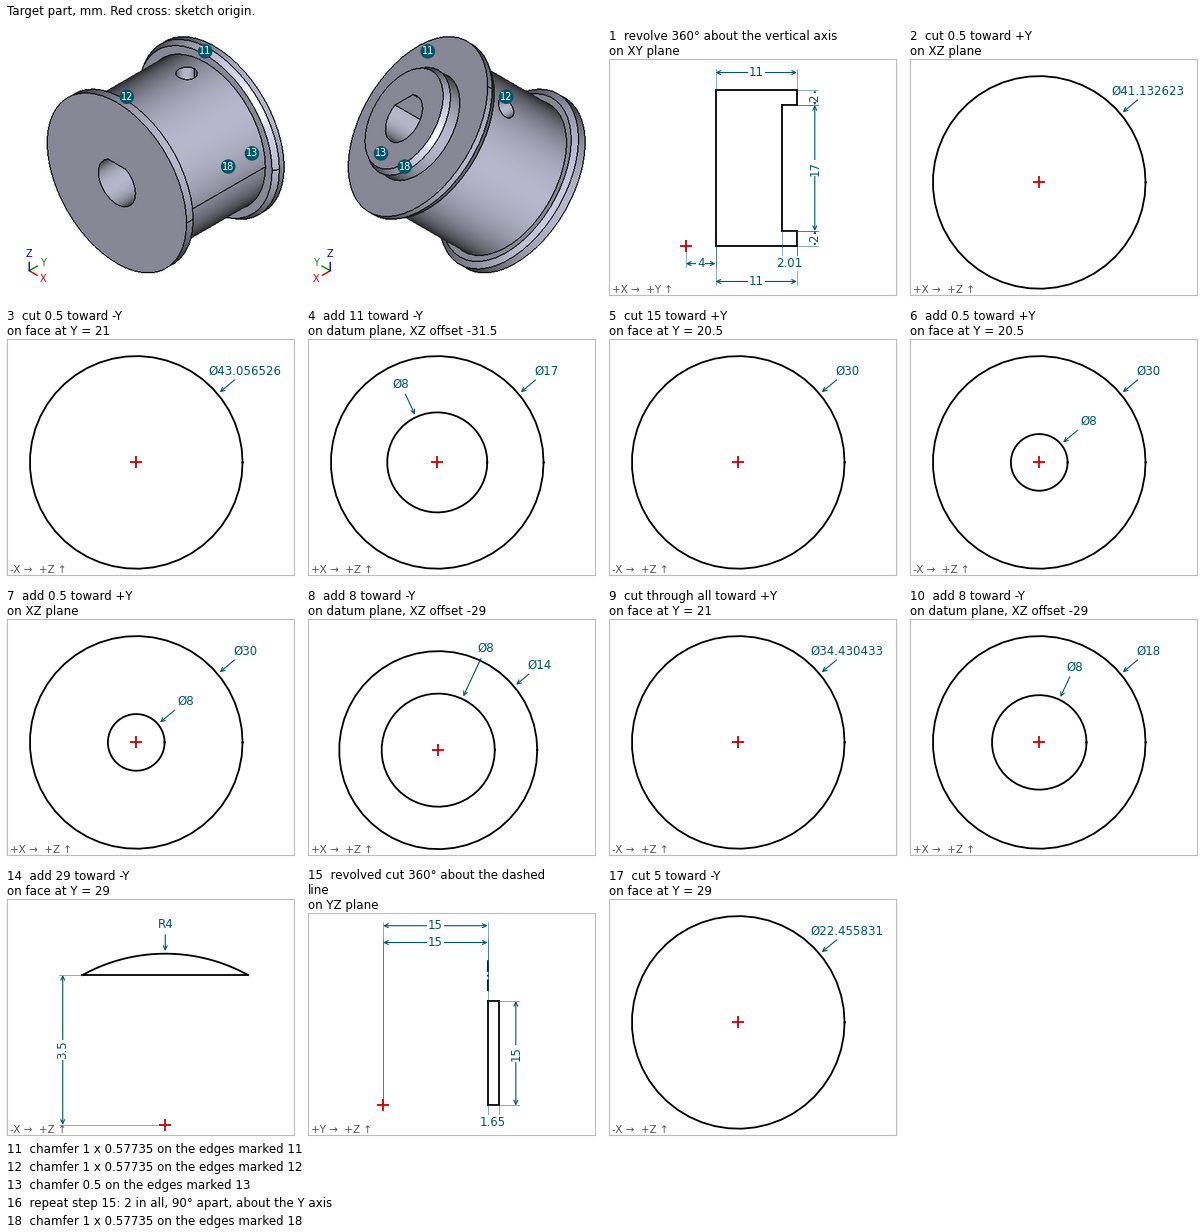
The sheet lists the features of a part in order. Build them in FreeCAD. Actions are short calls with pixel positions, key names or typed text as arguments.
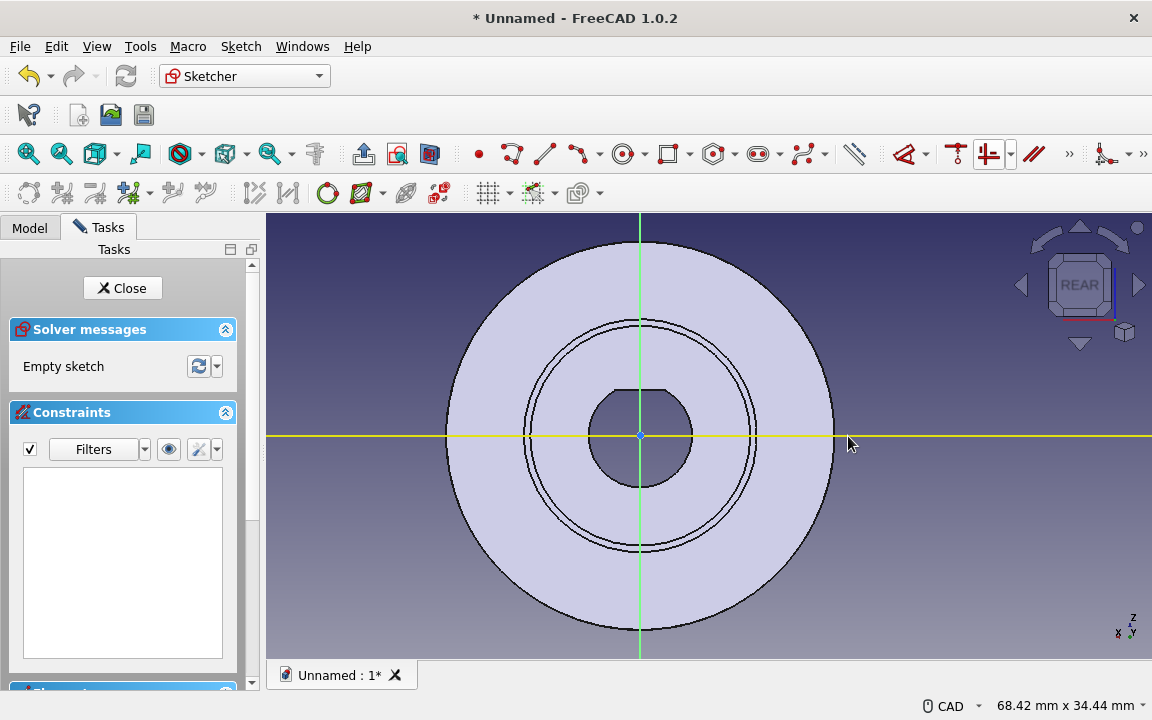
click(622, 154)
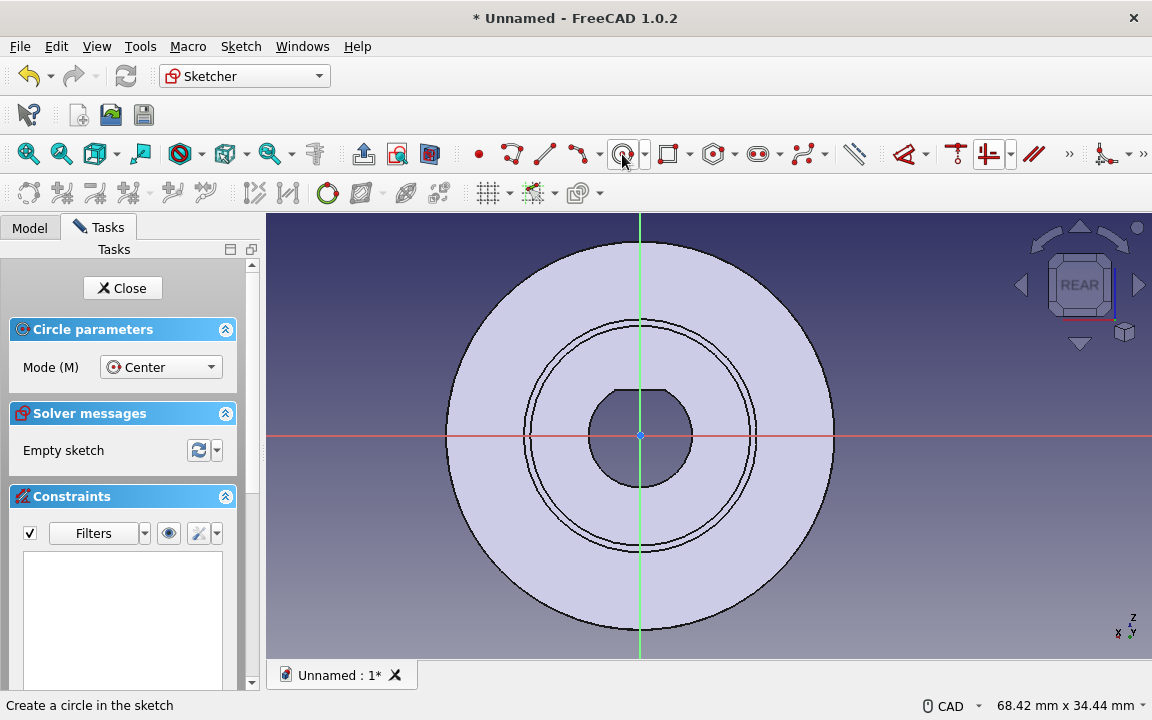
click(640, 436)
move(743, 333)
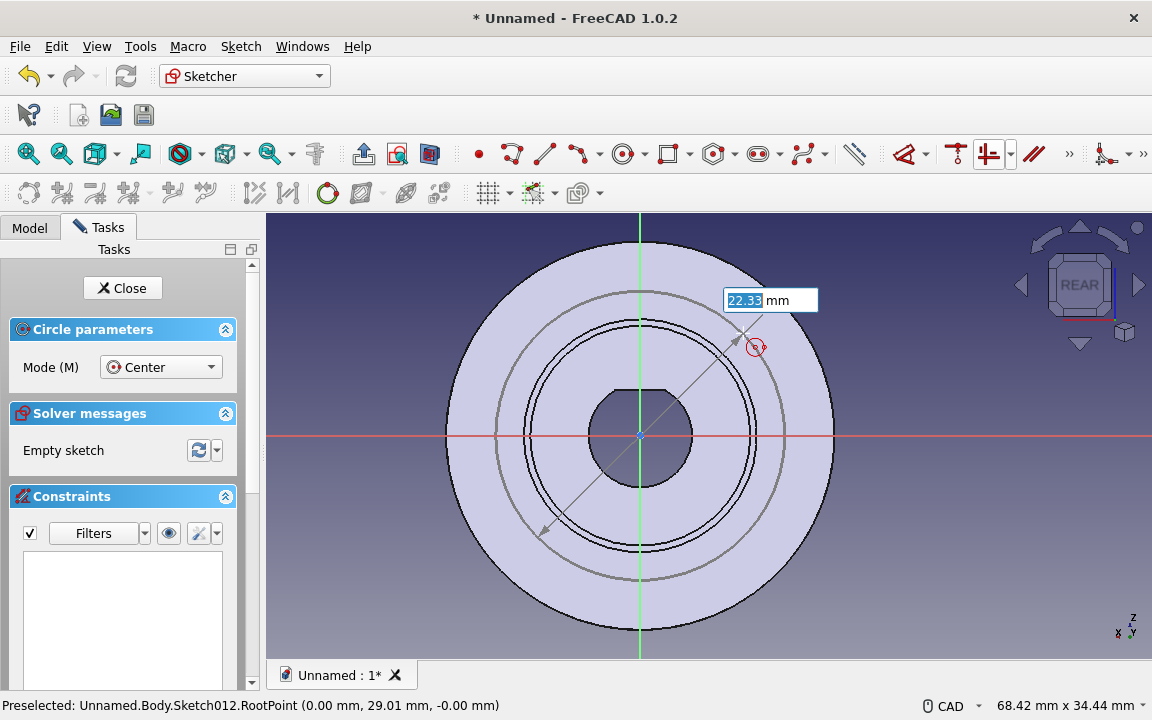
text(22.455831)
key(Return)
key(Escape)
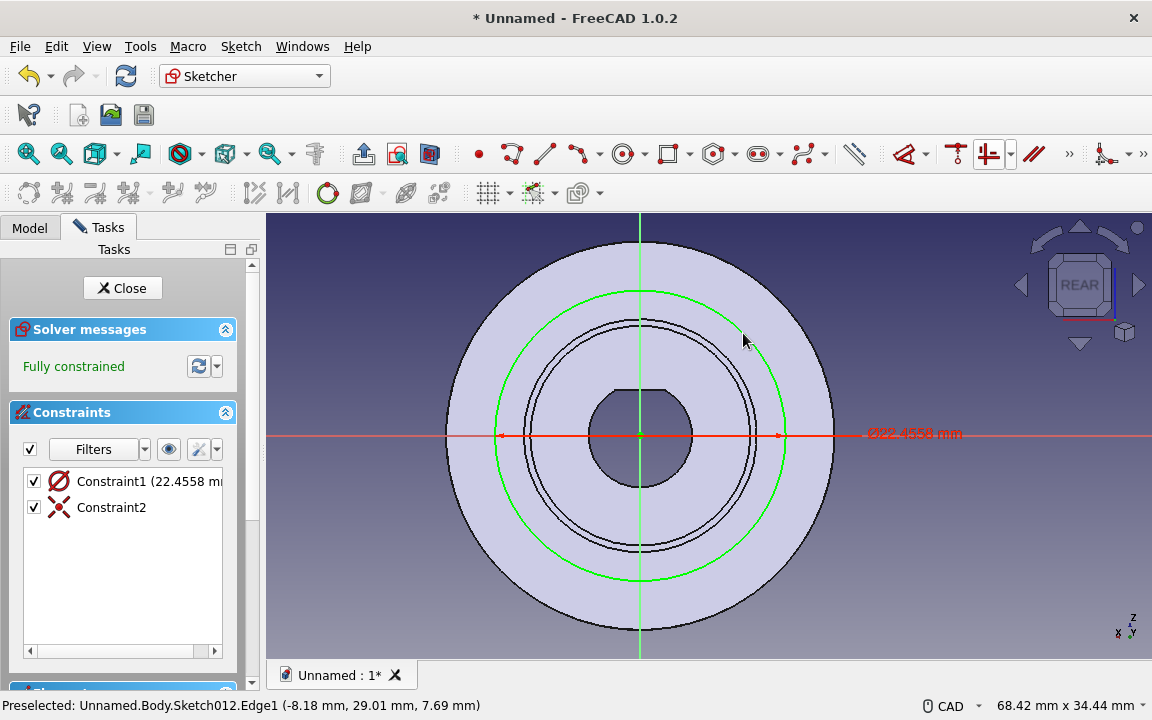
click(123, 288)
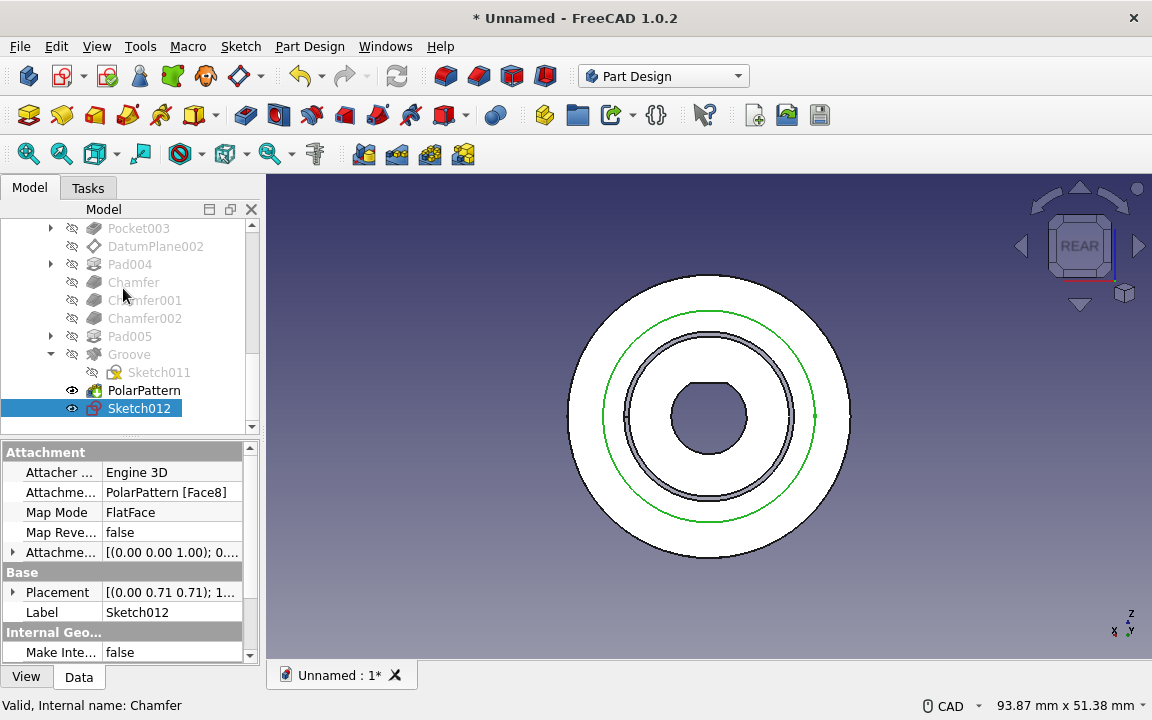
click(246, 116)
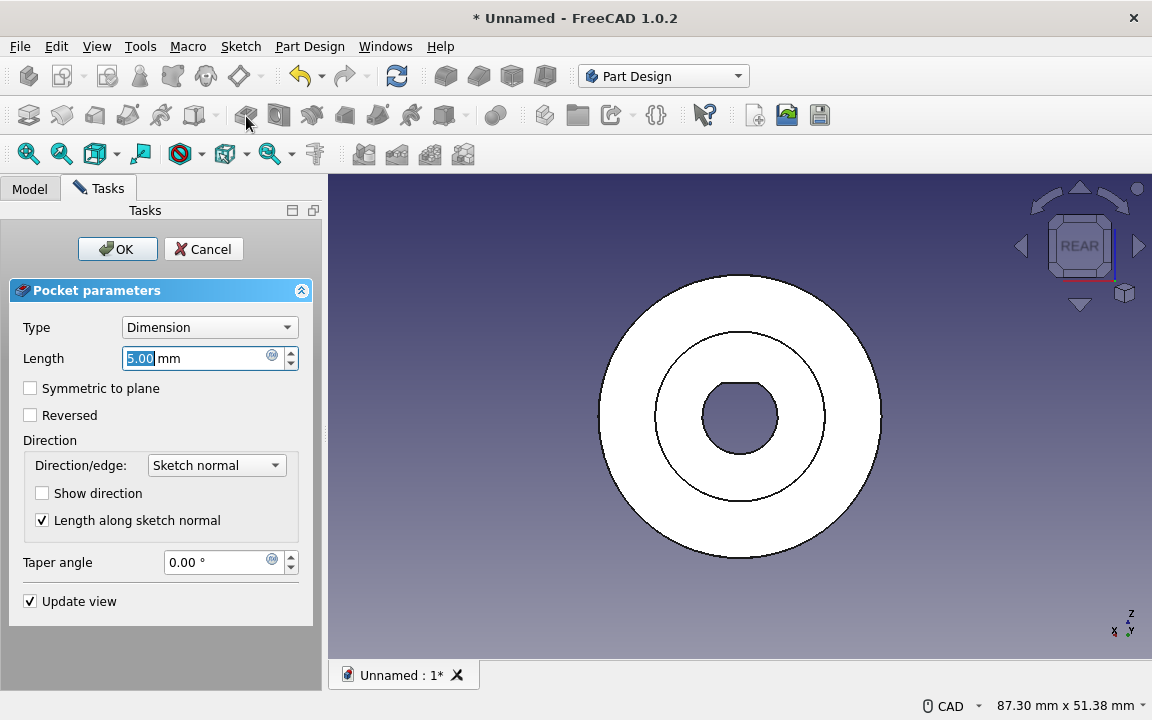
text(5)
key(Tab)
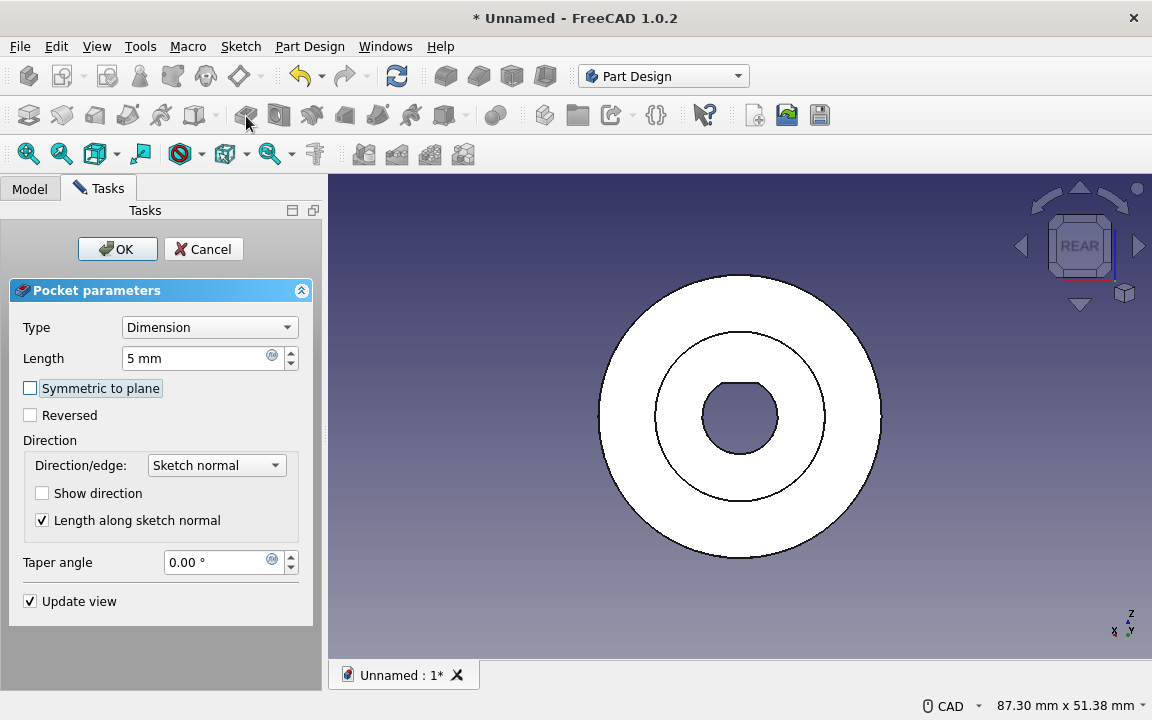
click(118, 249)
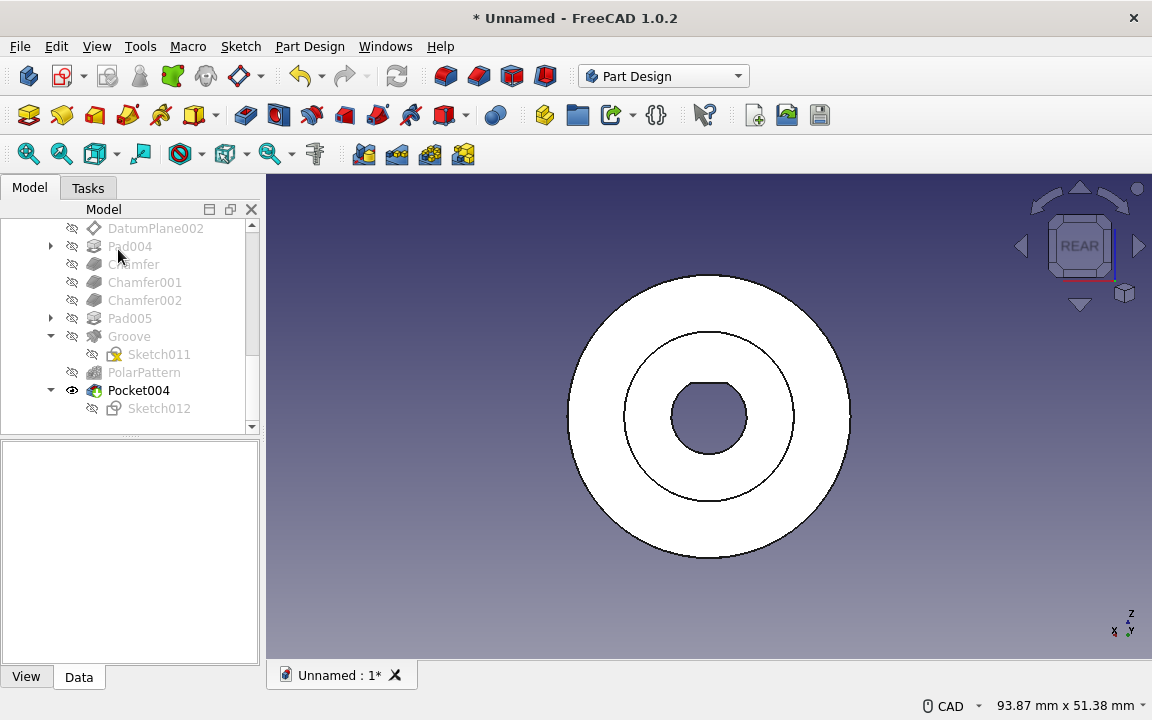
click(794, 415)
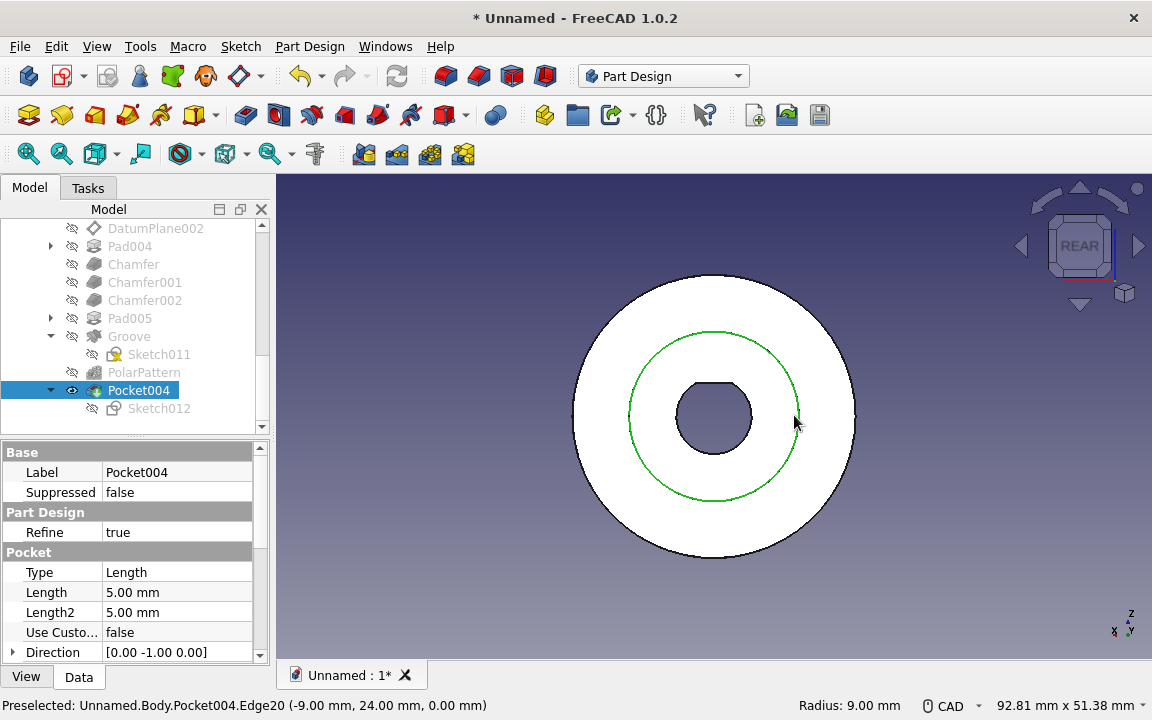
click(479, 76)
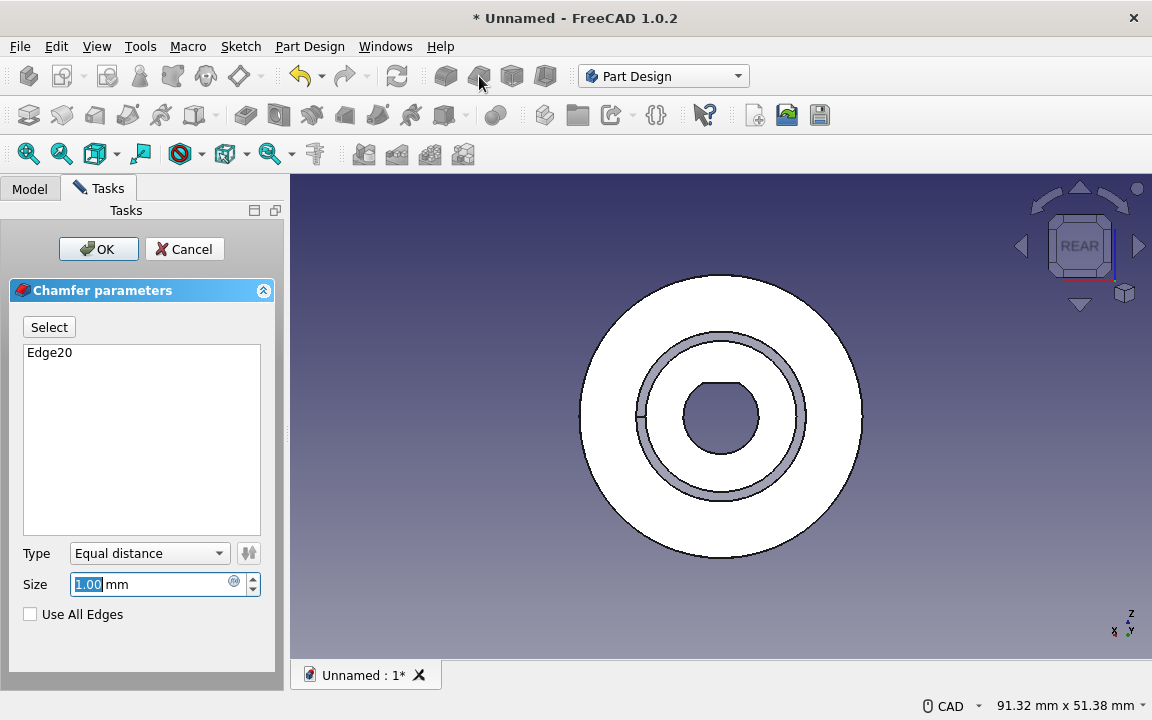
text(1)
key(Tab)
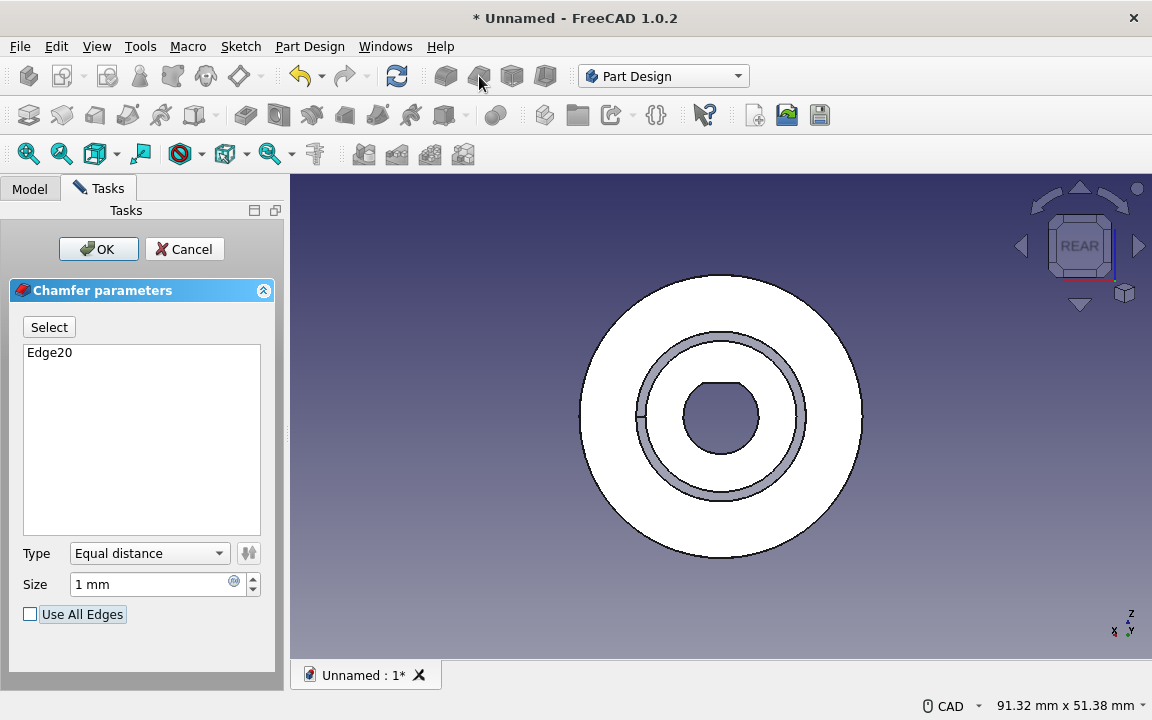
click(150, 554)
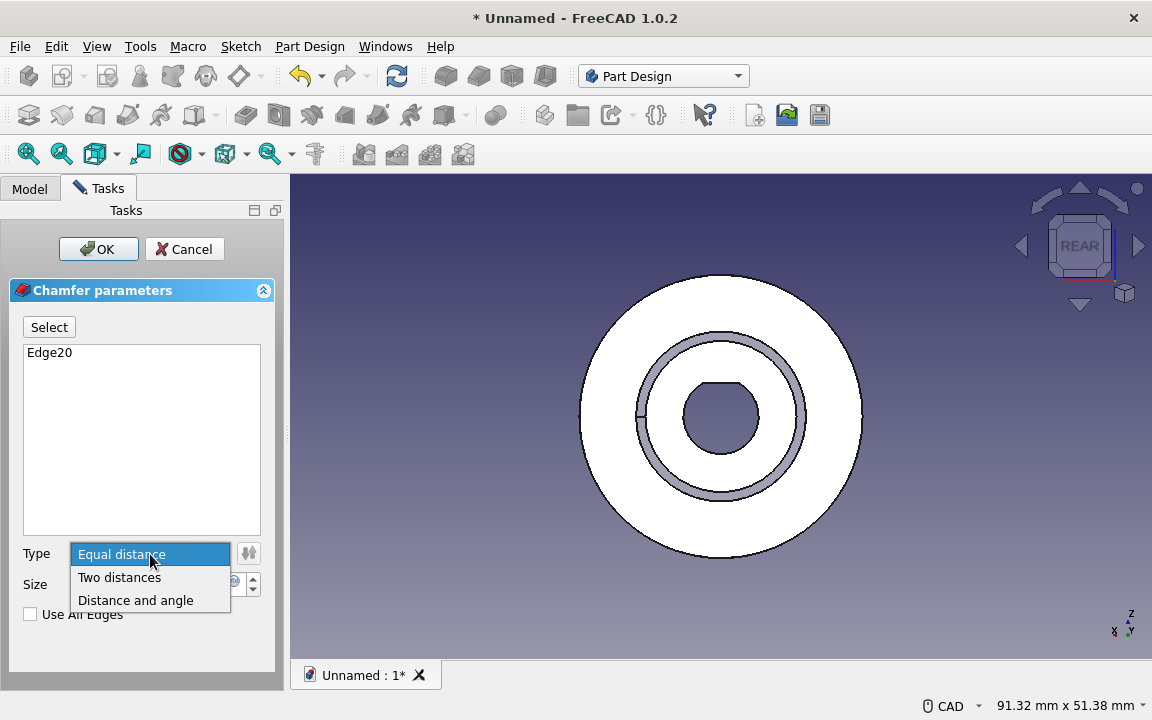
click(148, 578)